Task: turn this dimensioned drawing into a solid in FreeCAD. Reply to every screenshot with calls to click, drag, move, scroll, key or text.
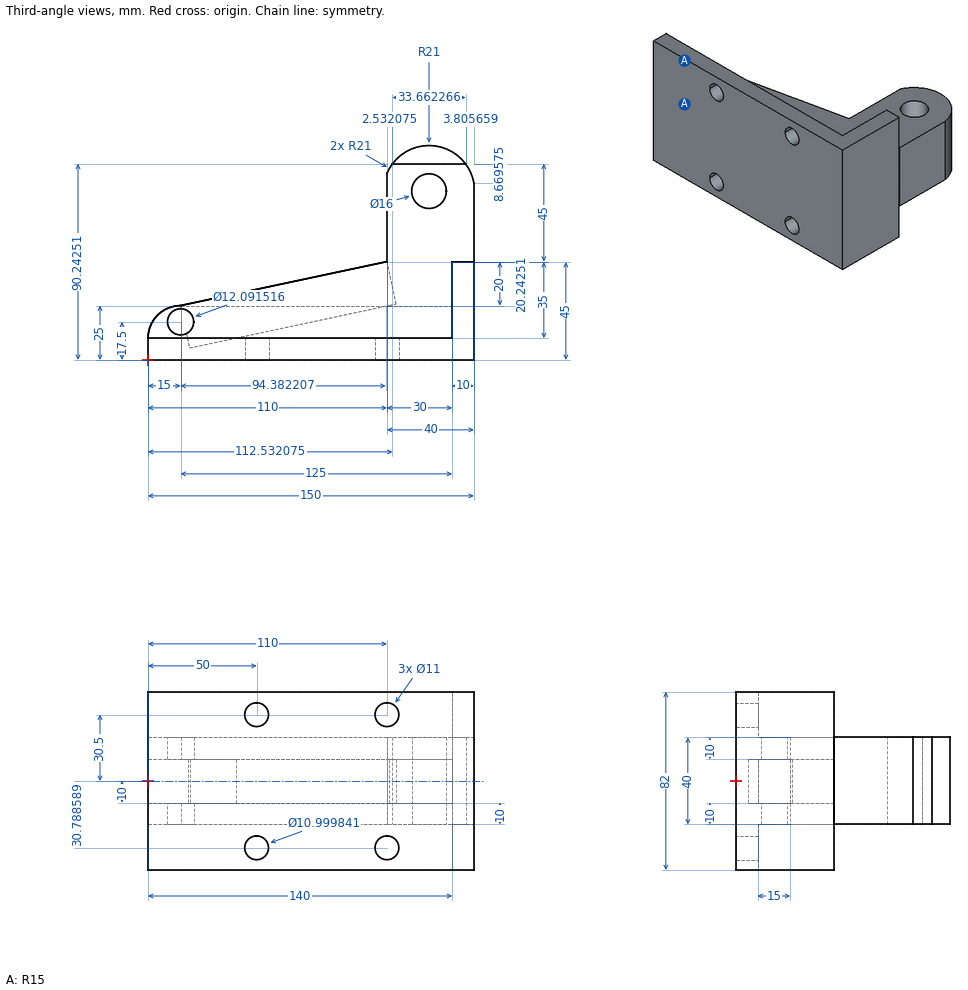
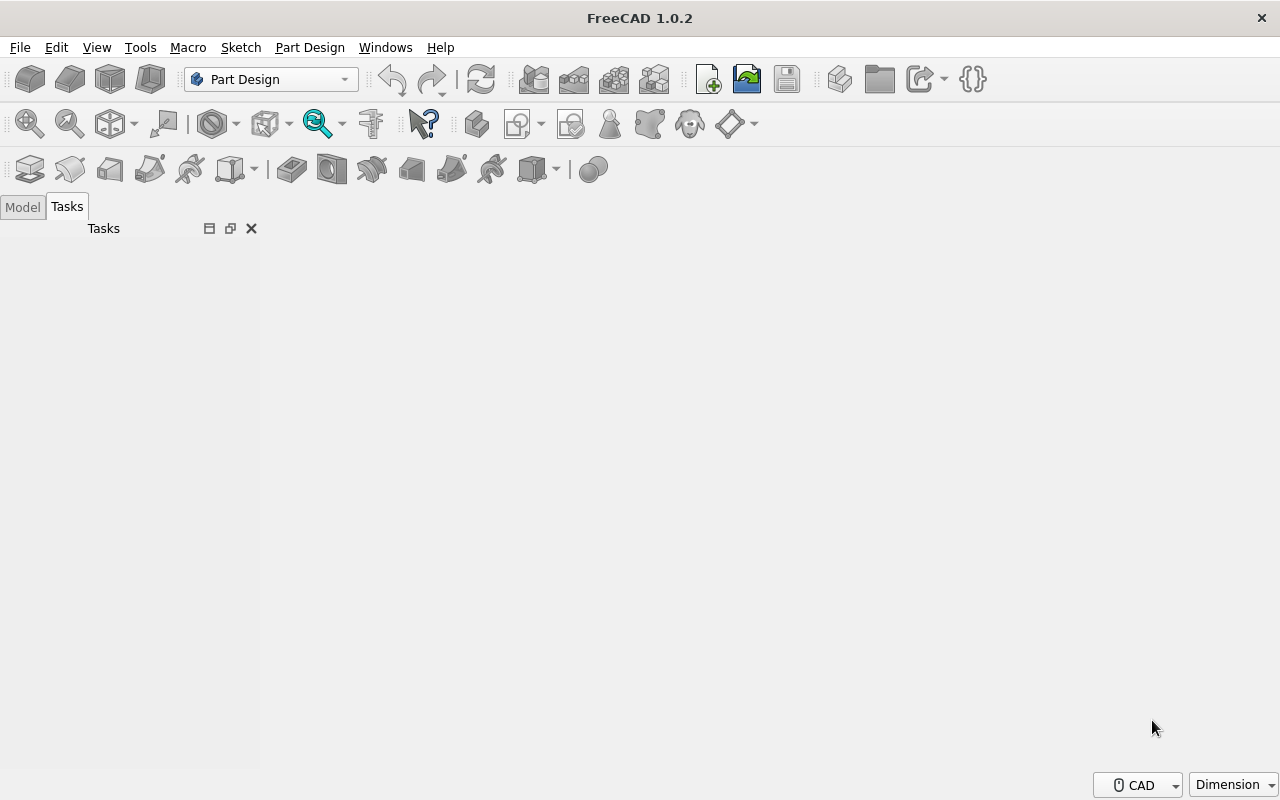
key(ctrl+n)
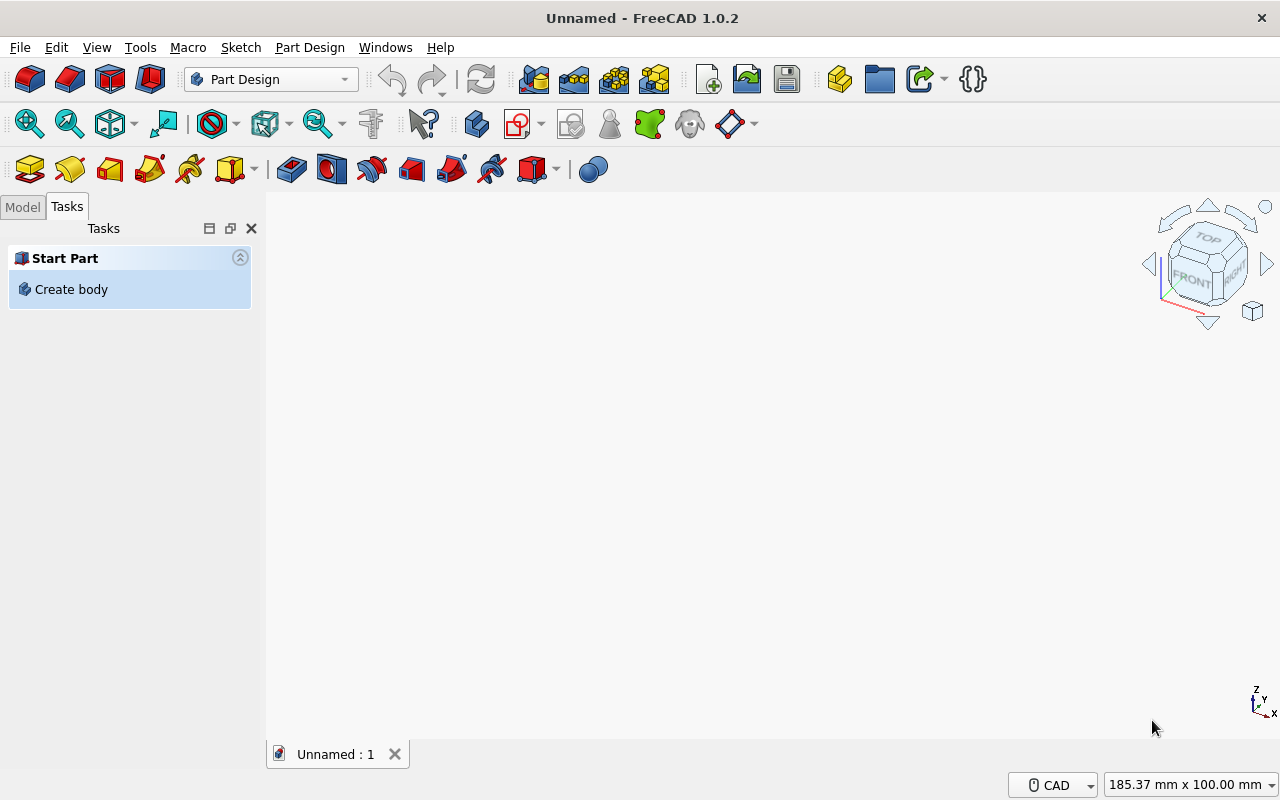
click(518, 124)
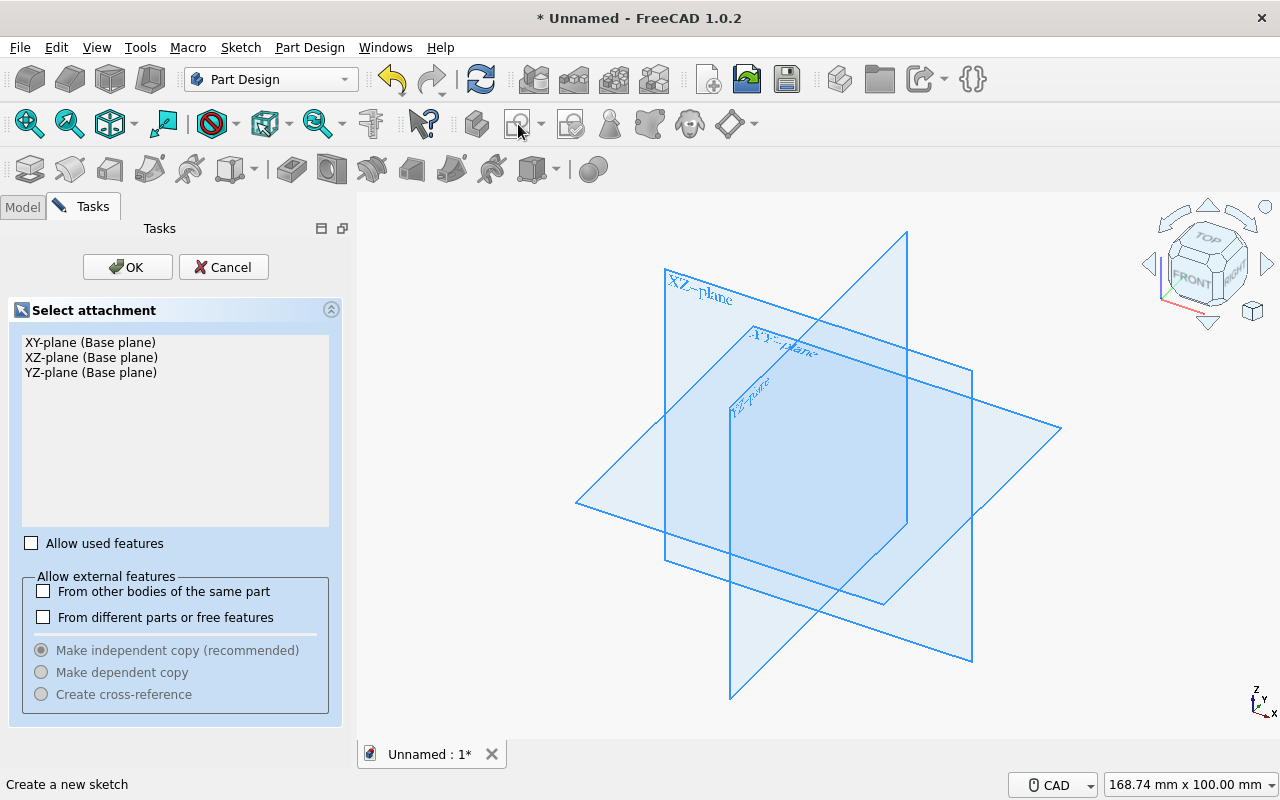
click(82, 342)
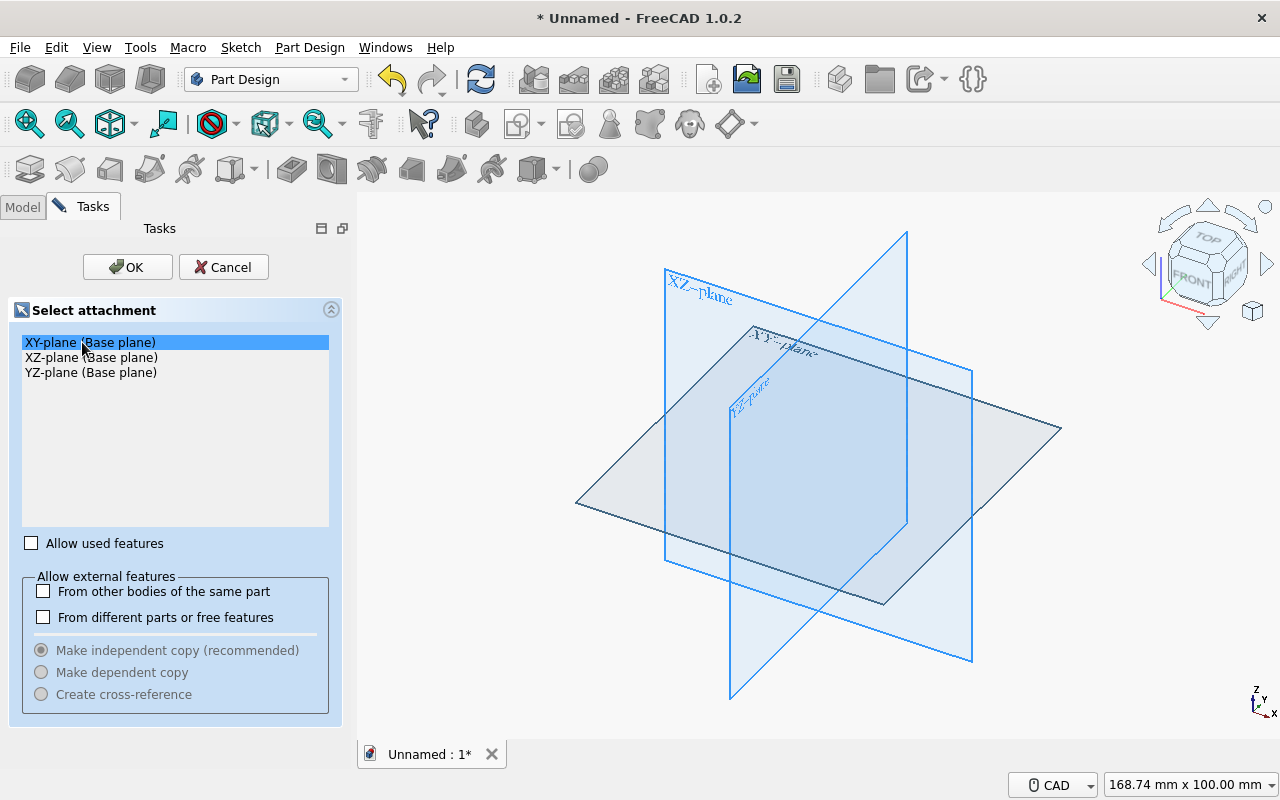
click(128, 267)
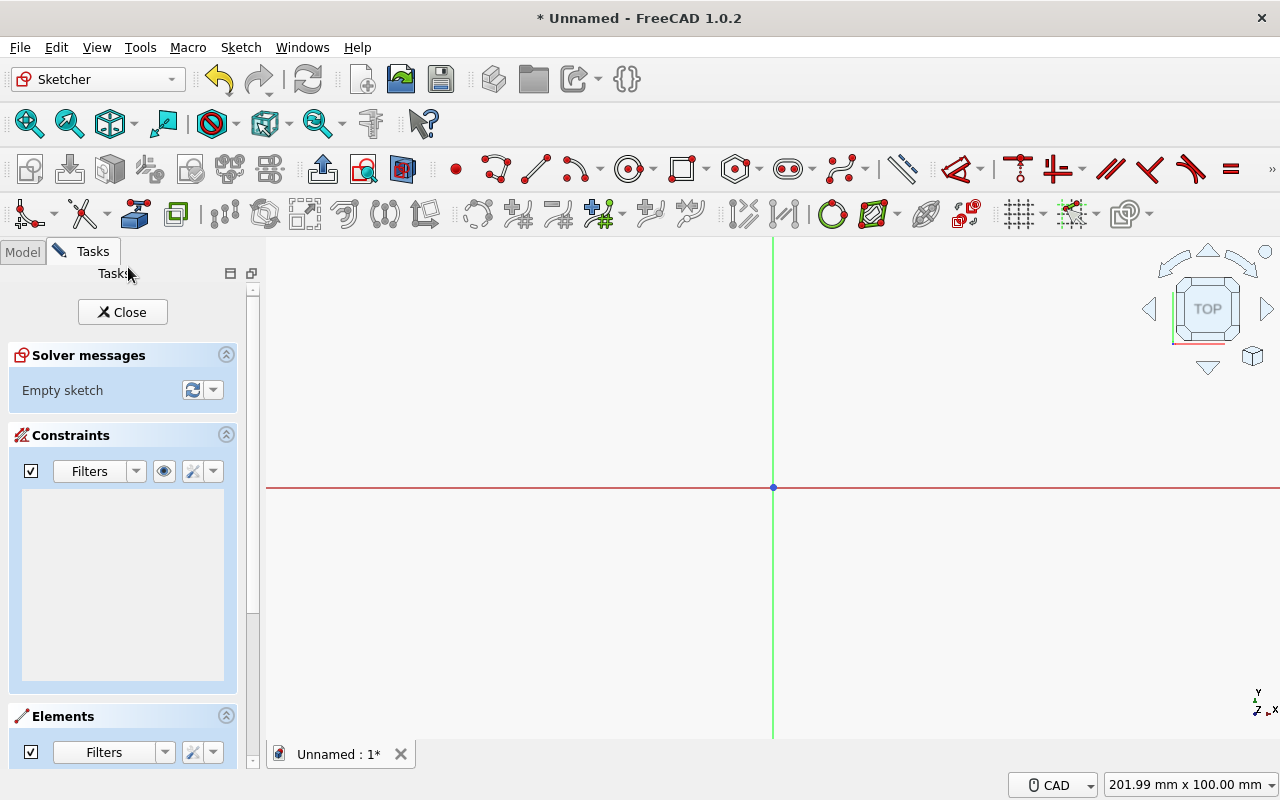
scroll(294, 625, down, 3)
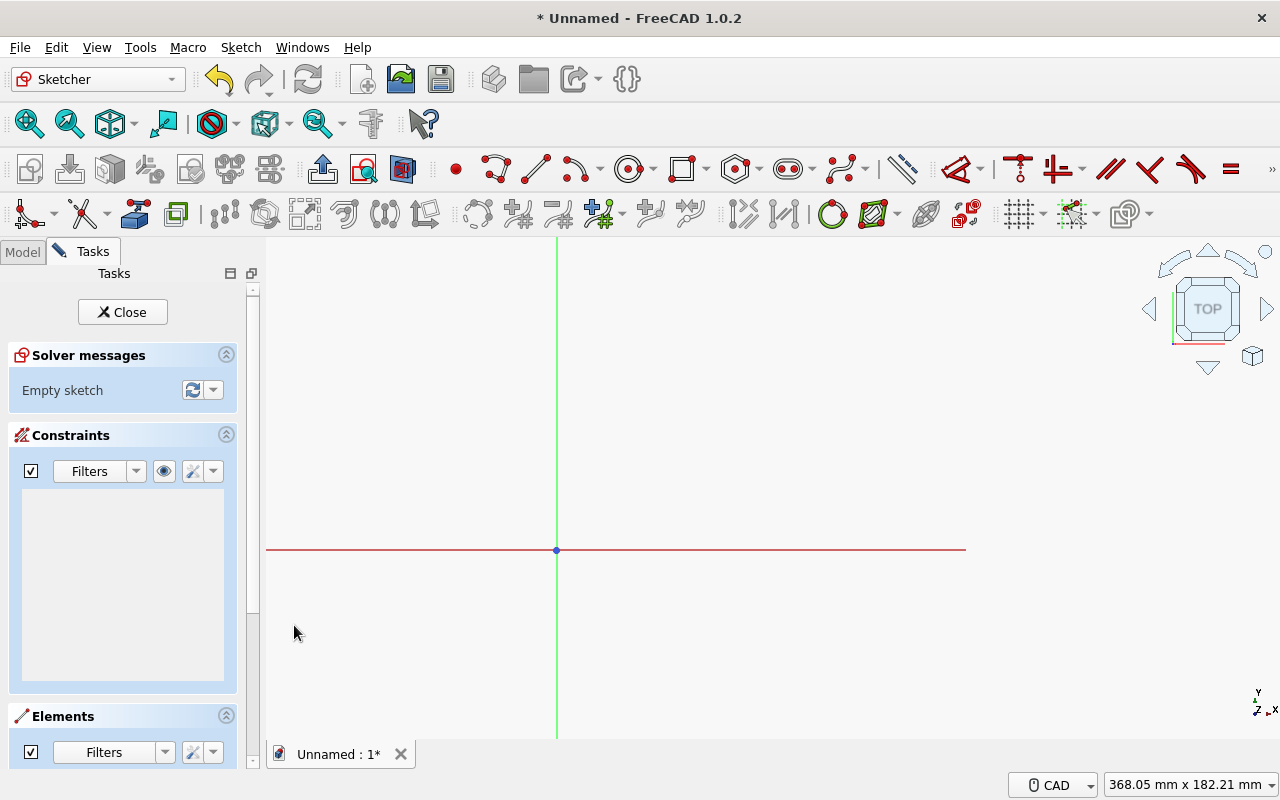
scroll(884, 489, up, 2)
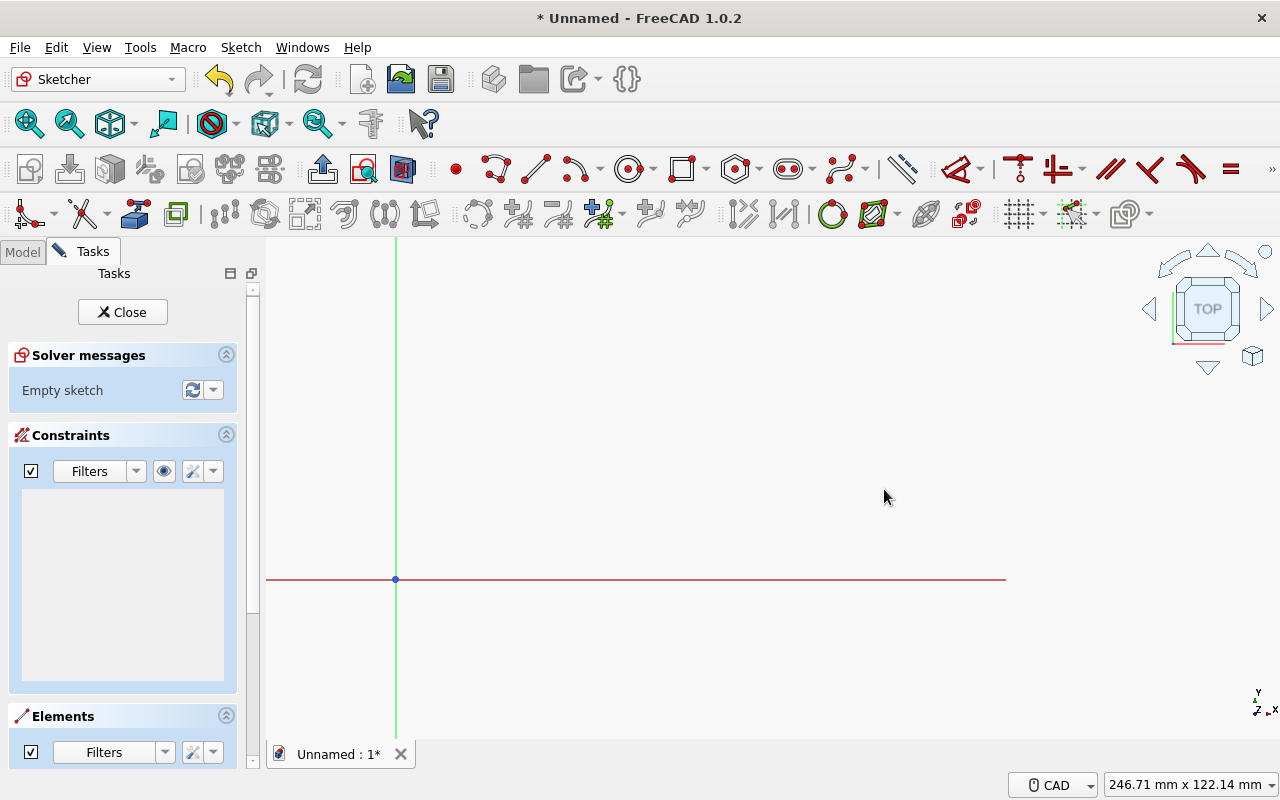
click(496, 170)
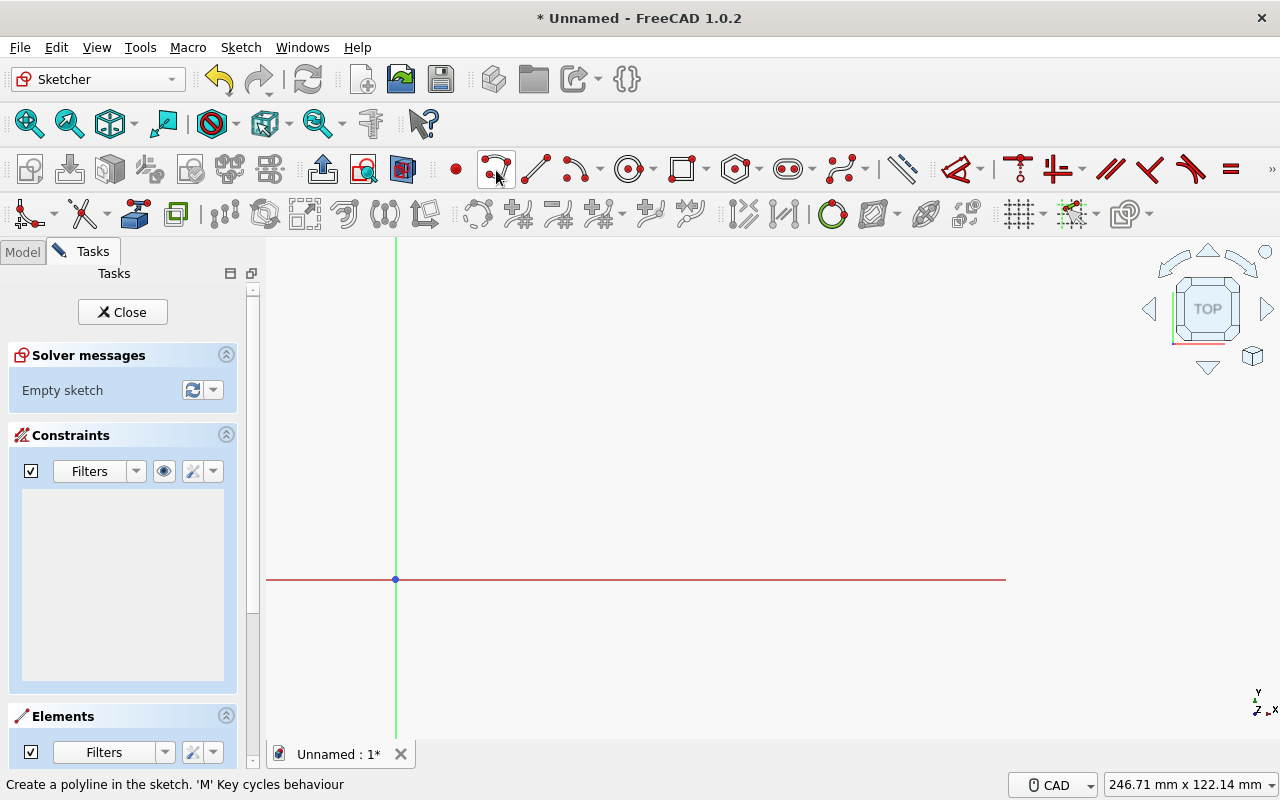
click(396, 580)
click(1012, 571)
click(1012, 395)
click(971, 395)
click(971, 539)
click(405, 539)
click(396, 580)
key(Escape)
key(Escape)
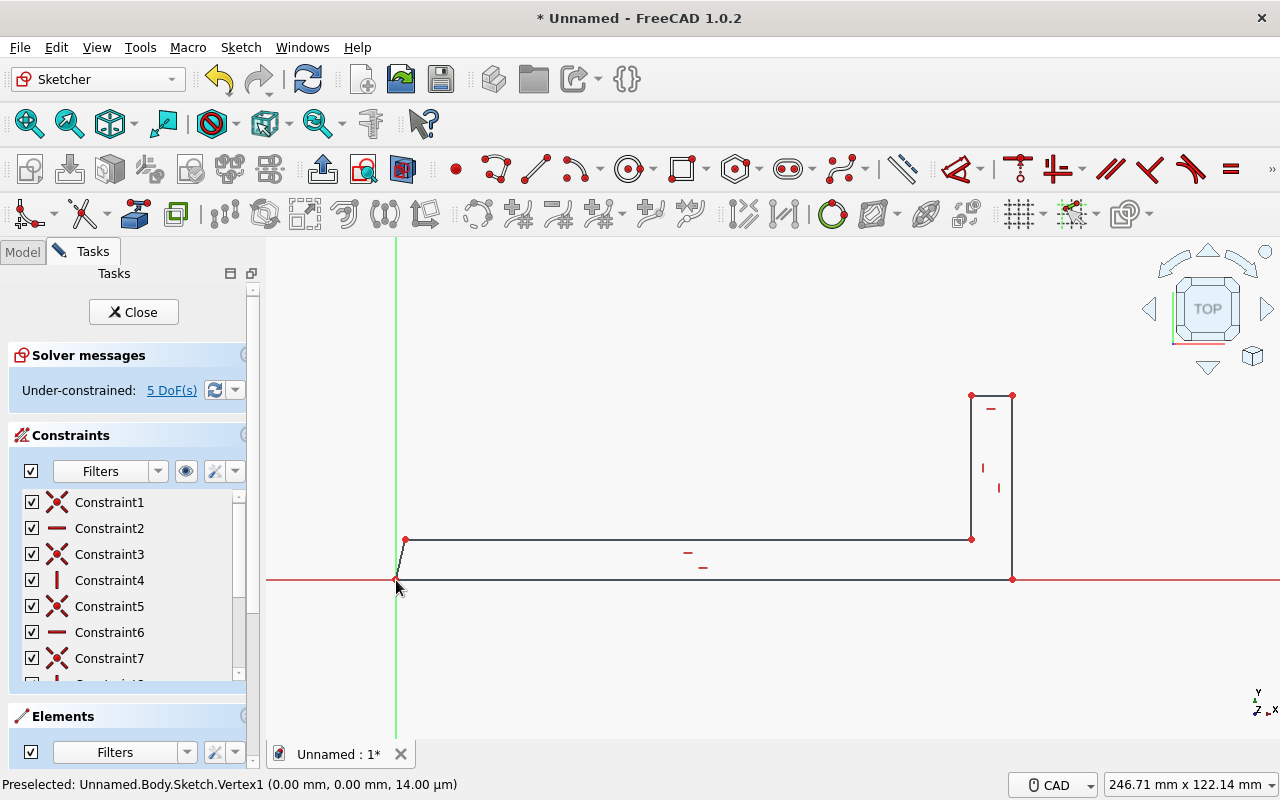
click(398, 568)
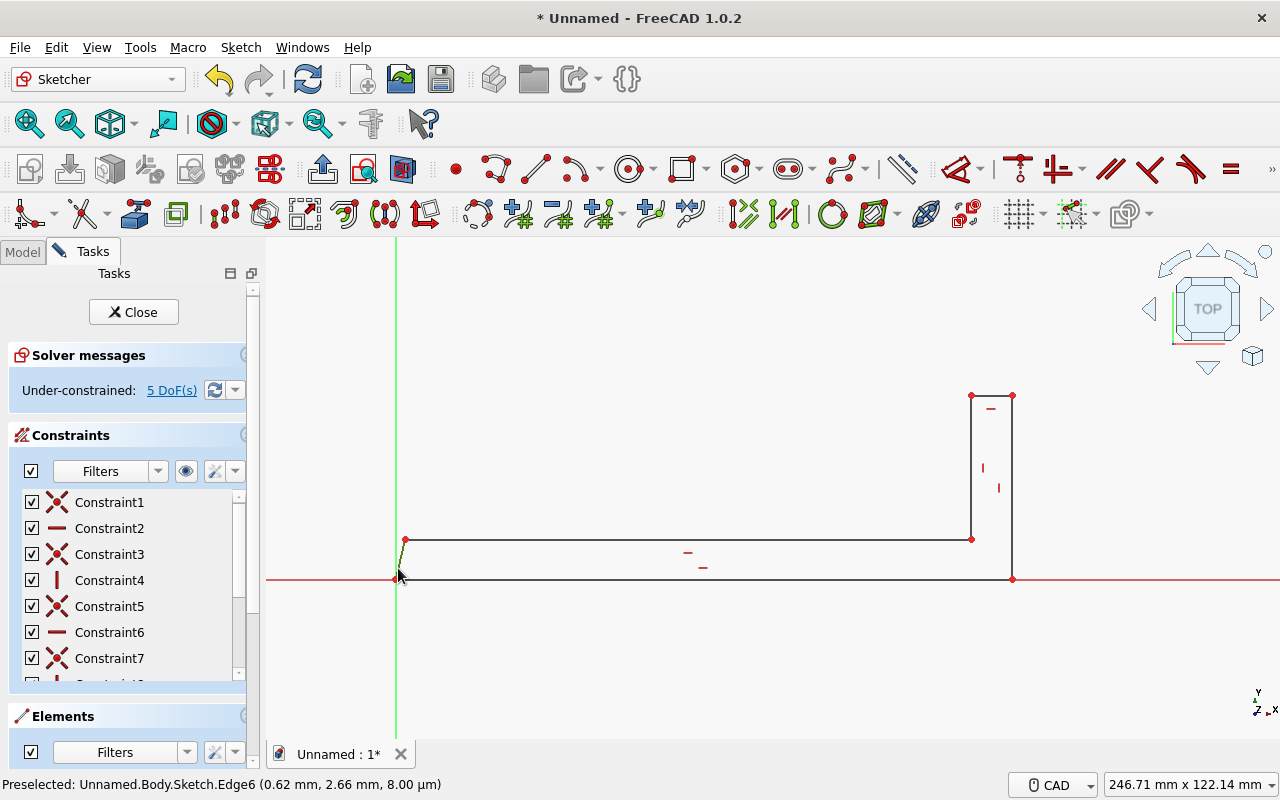
click(1084, 170)